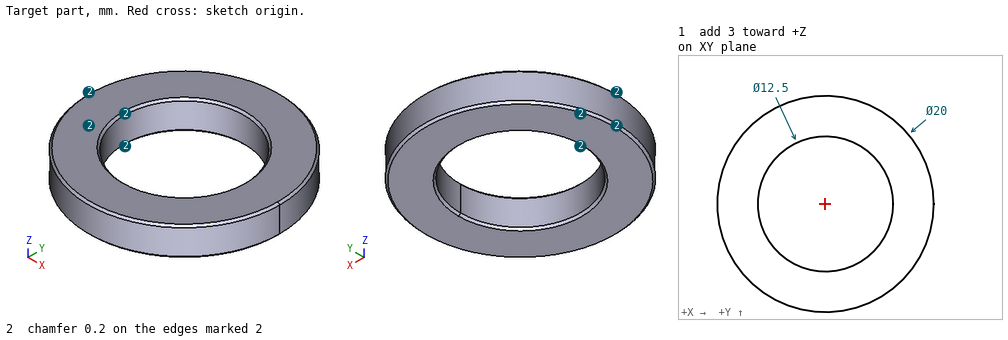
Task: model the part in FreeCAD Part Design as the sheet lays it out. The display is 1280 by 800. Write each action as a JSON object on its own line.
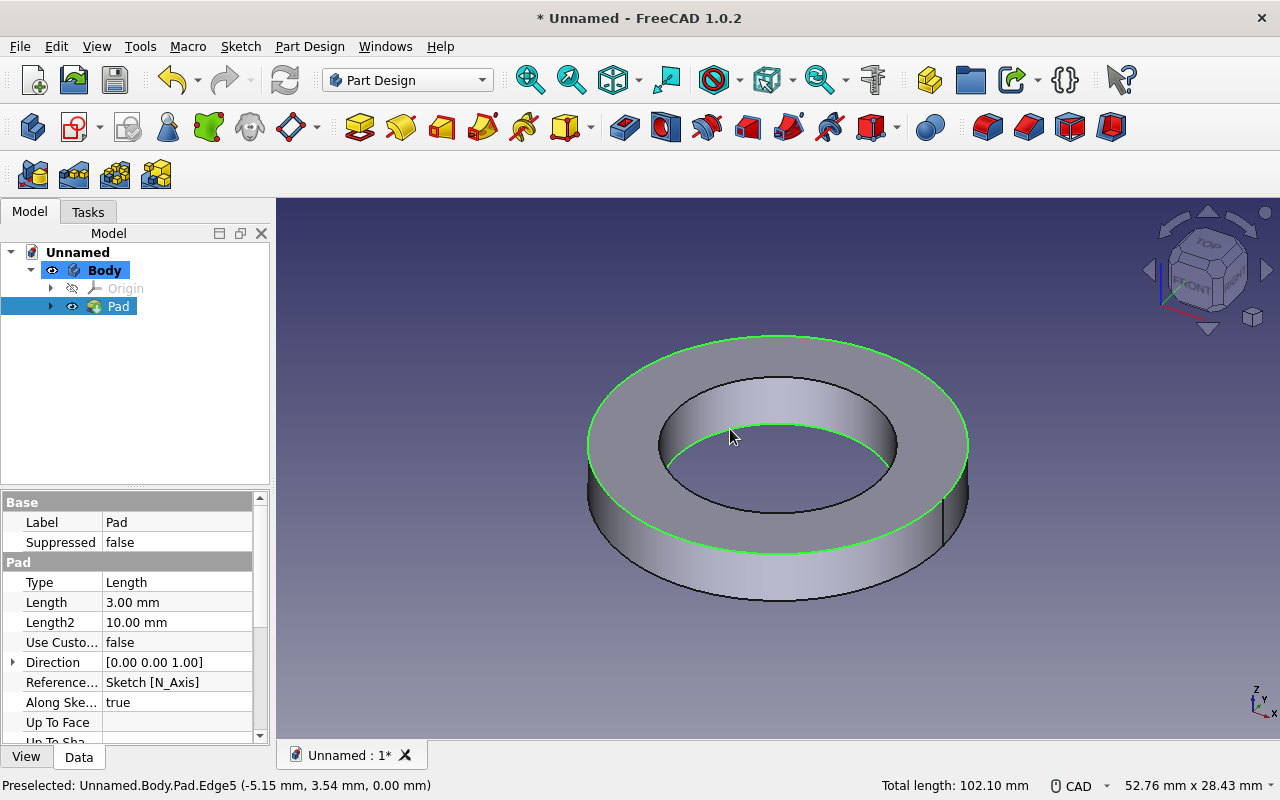
{"action": "left_click", "coordinate": [675, 410], "text": "ctrl"}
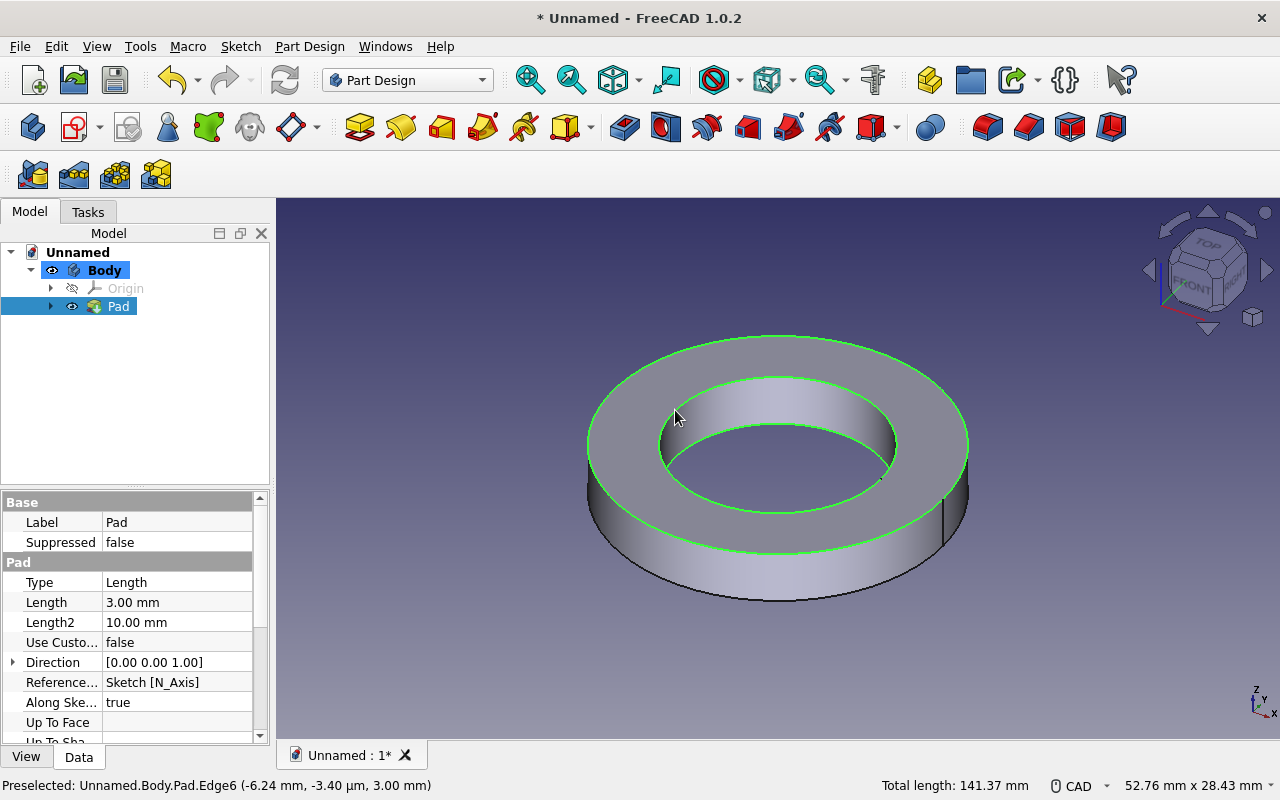
{"action": "key", "text": "0"}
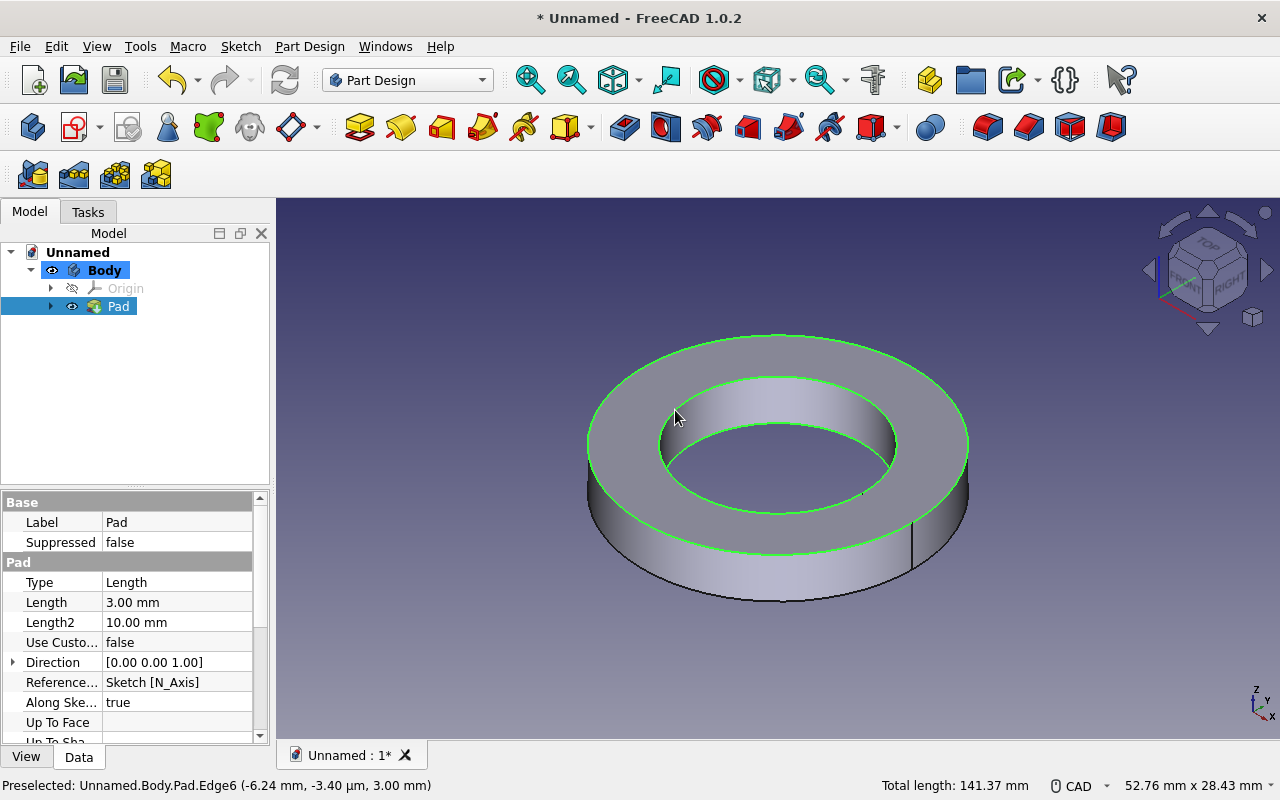
{"action": "key", "text": "2"}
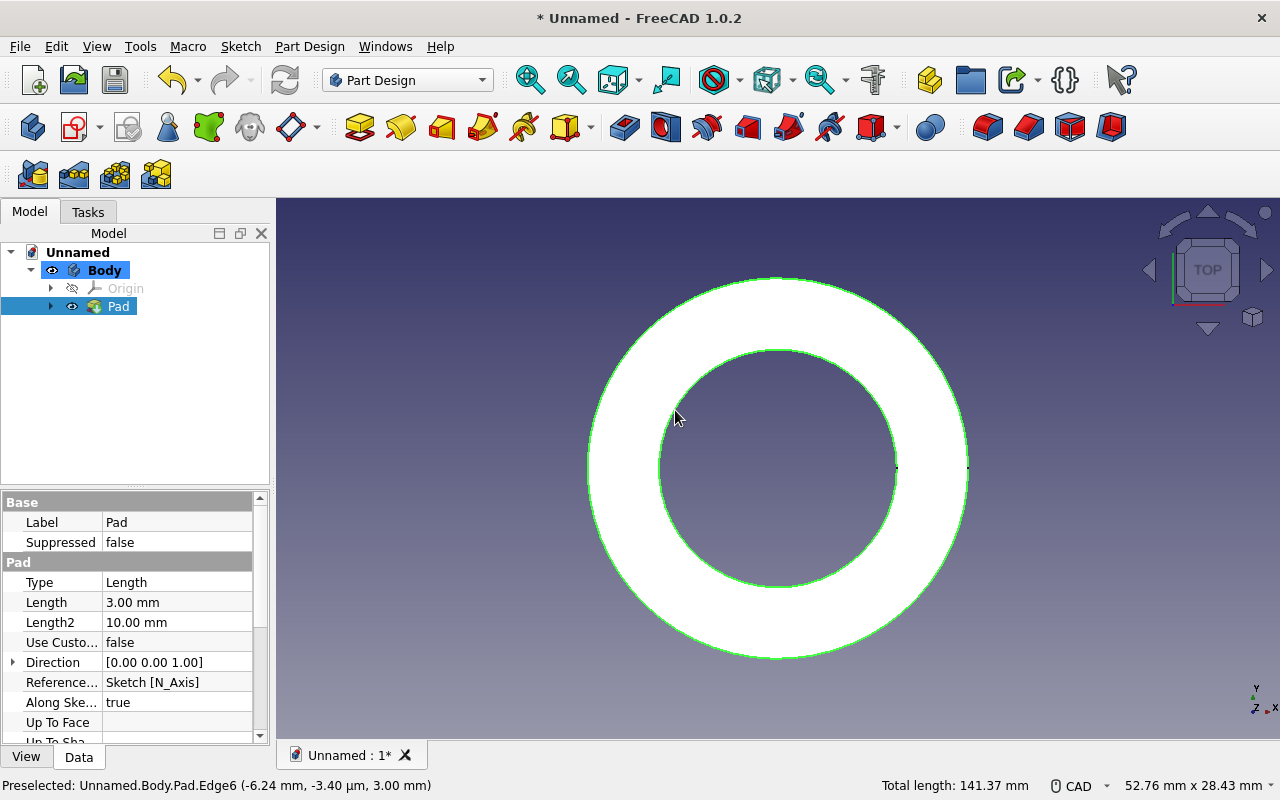
{"action": "key", "text": "1"}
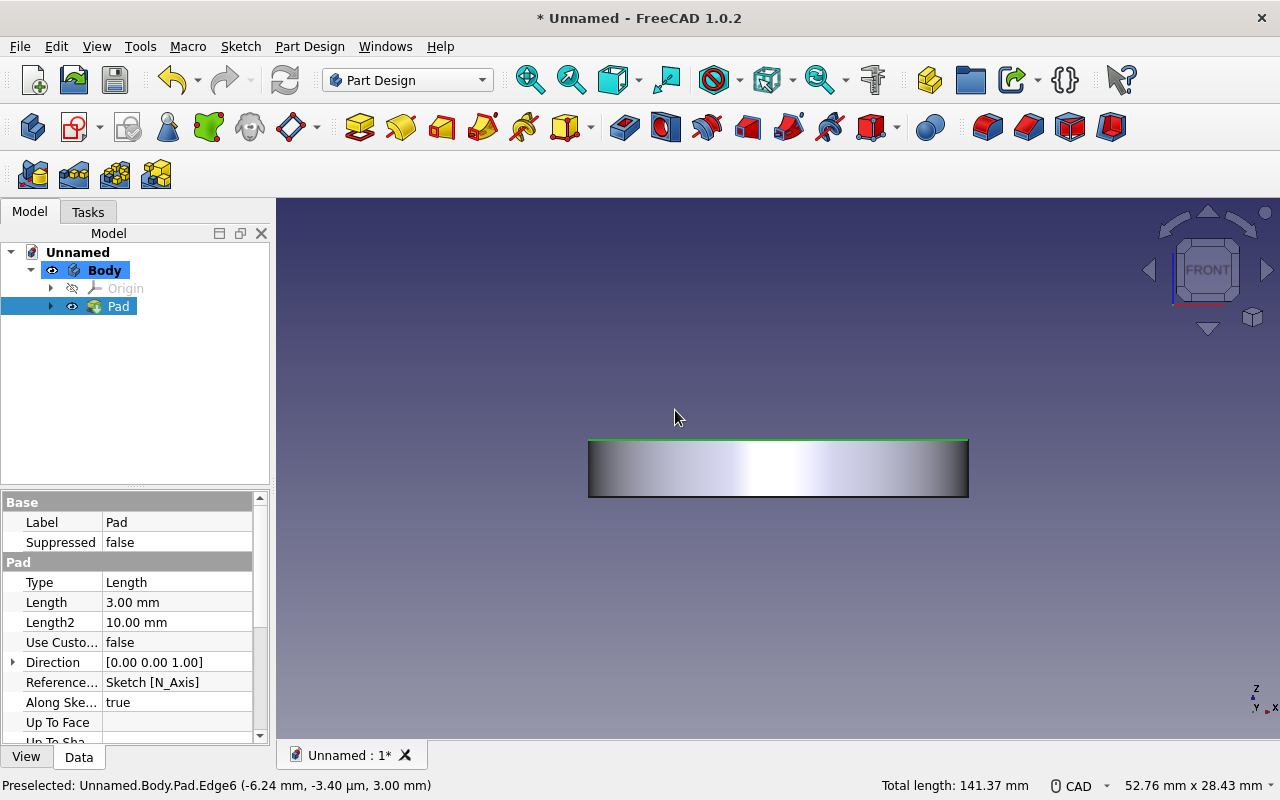
{"action": "left_click", "coordinate": [531, 80]}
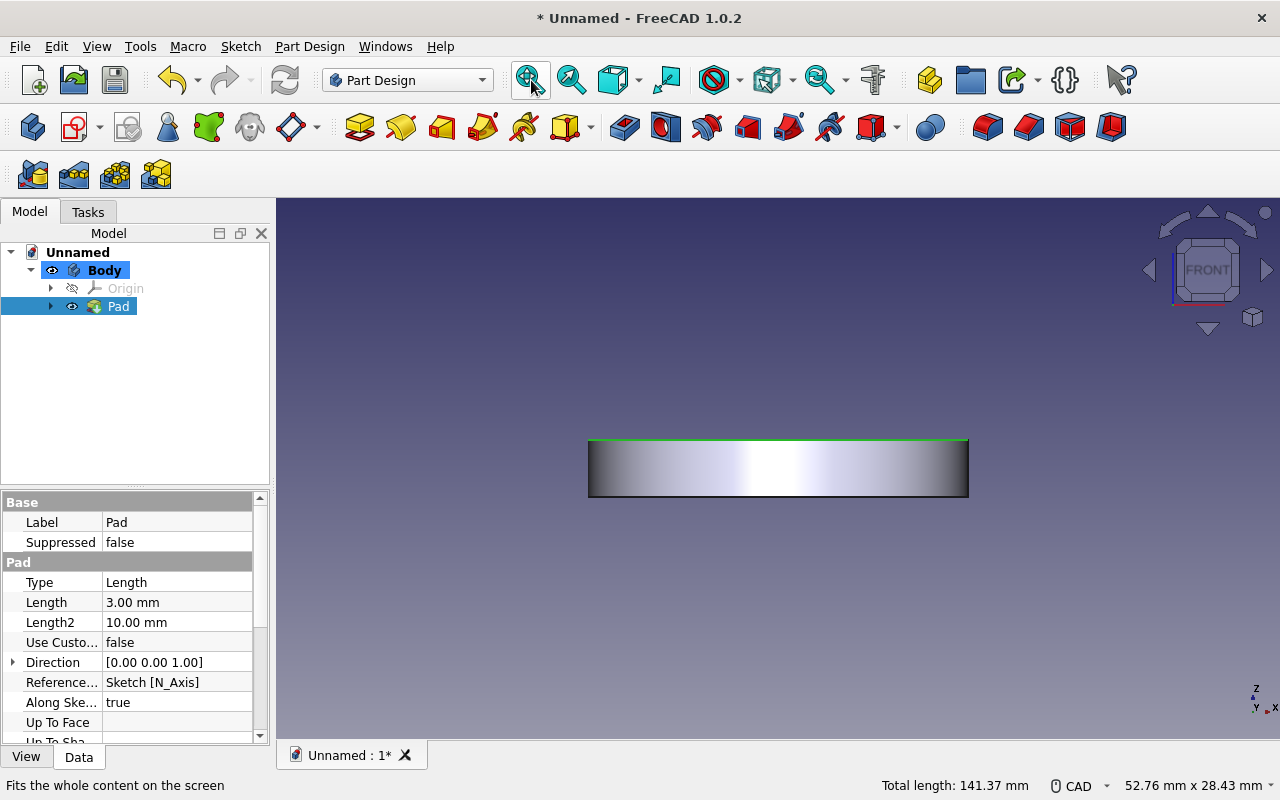
{"action": "left_click", "coordinate": [624, 496], "text": "ctrl"}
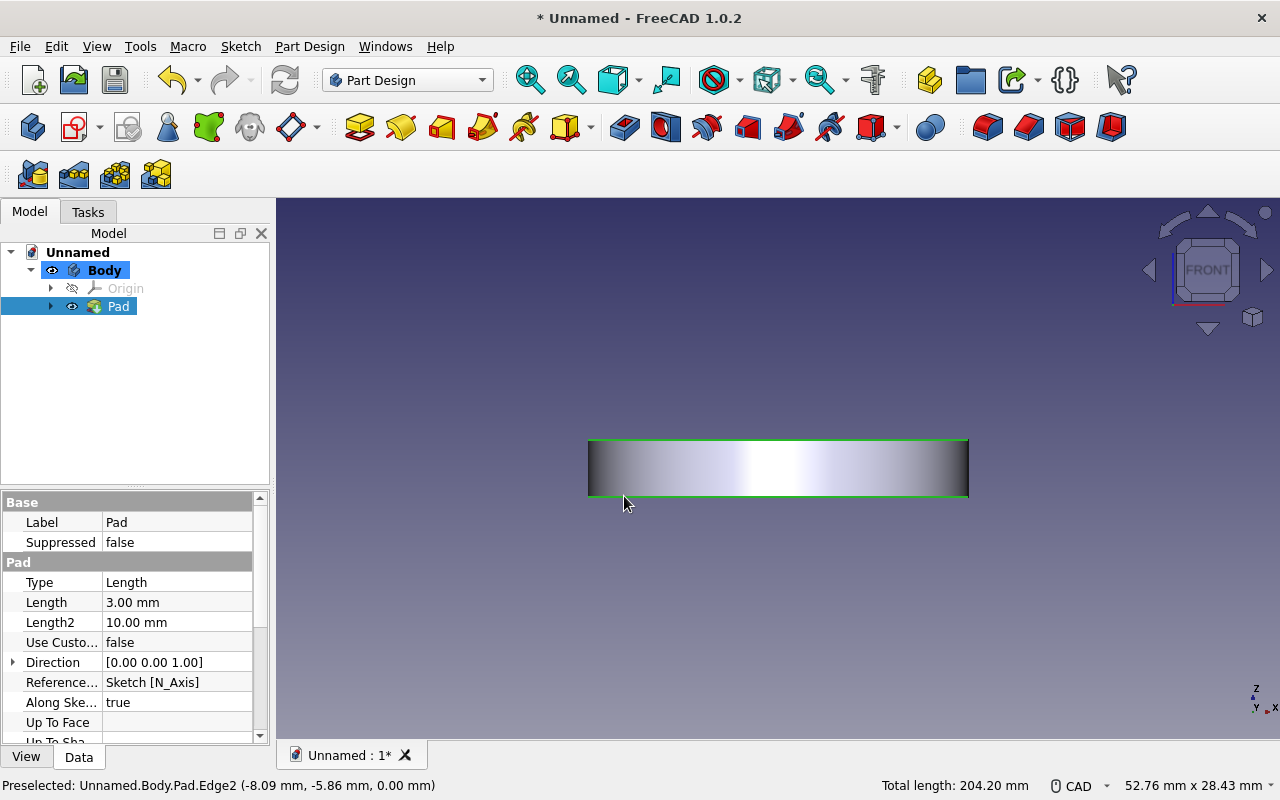
{"action": "left_click", "coordinate": [1029, 128]}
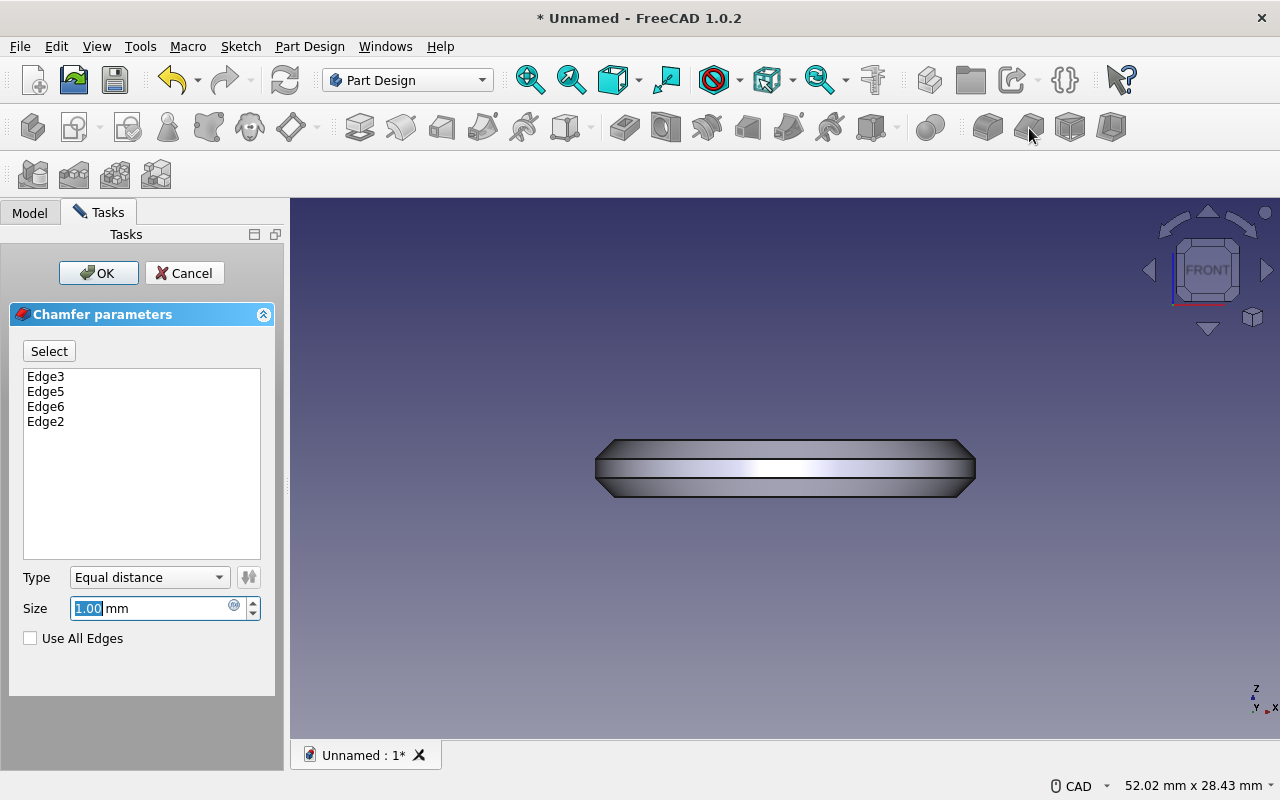
{"action": "type", "text": "0.2"}
{"action": "key", "text": "Tab"}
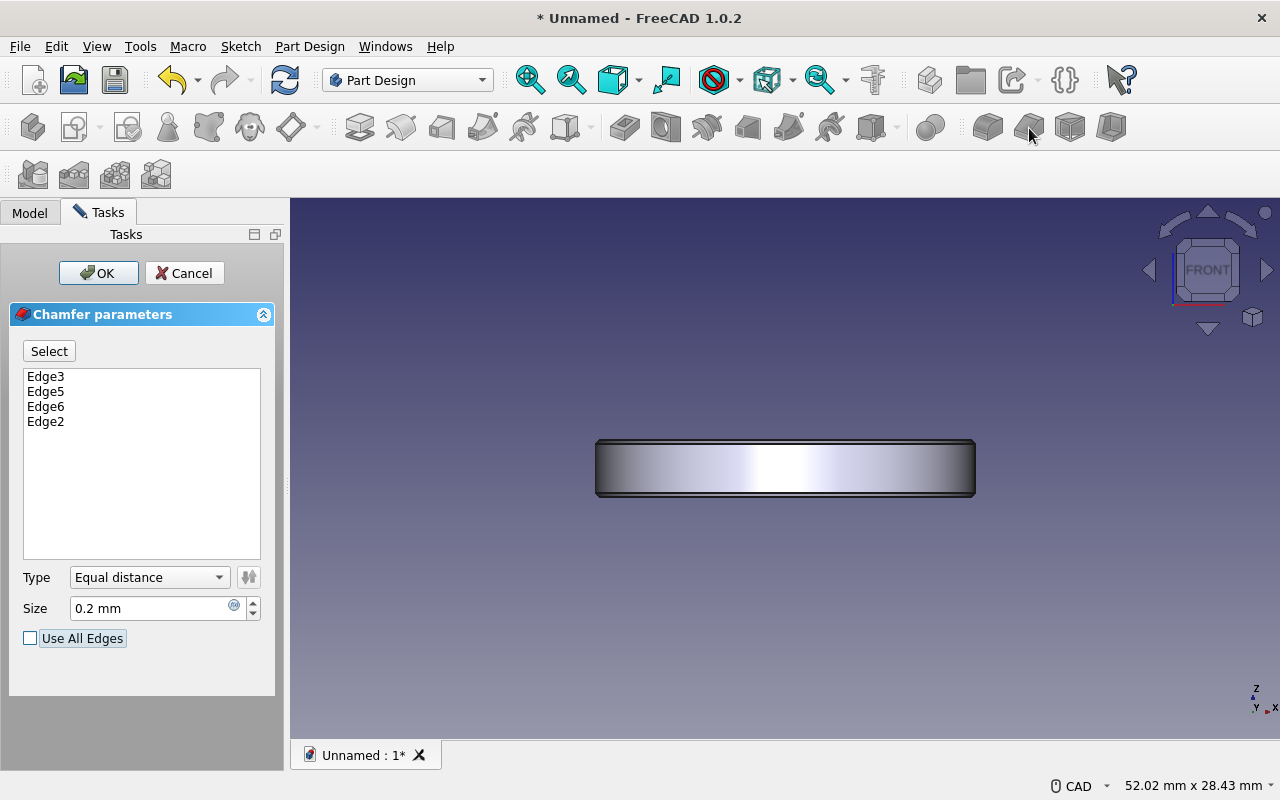
{"action": "left_click", "coordinate": [99, 273]}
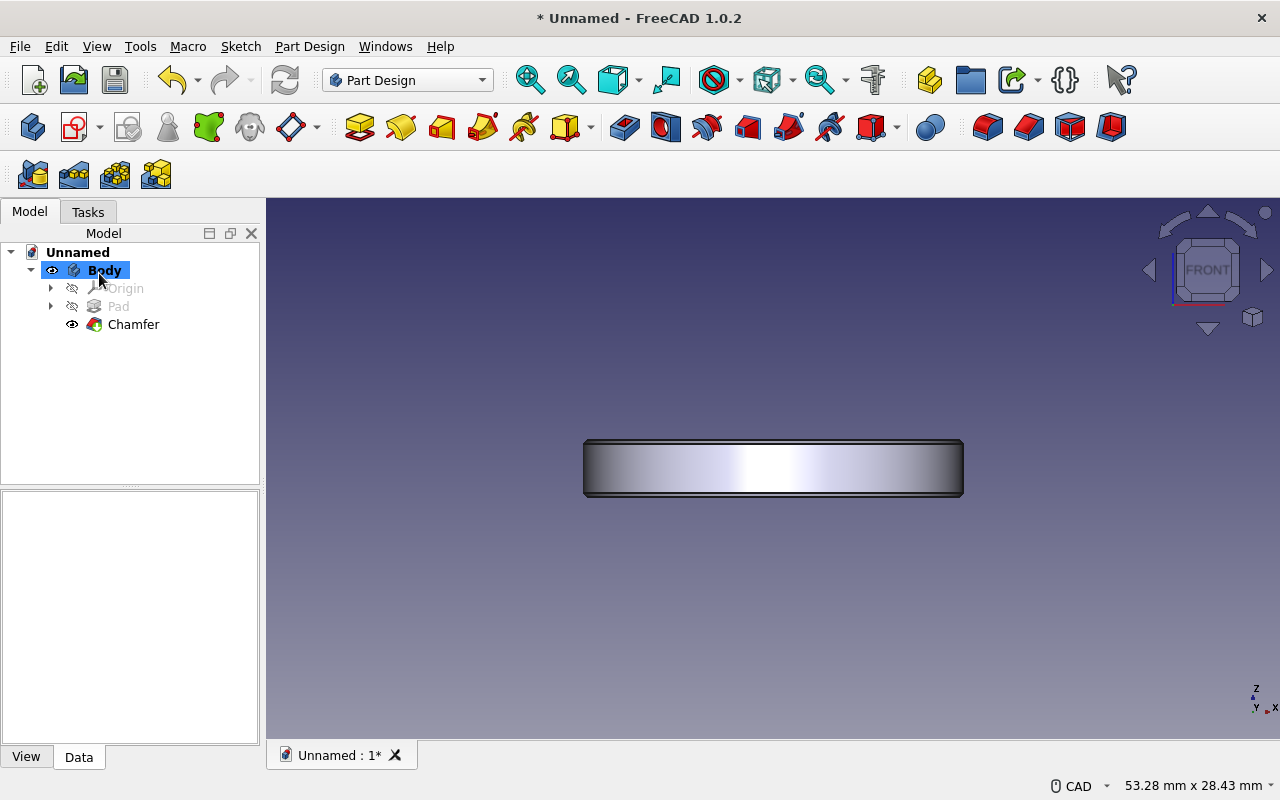
{"action": "key", "text": "0"}